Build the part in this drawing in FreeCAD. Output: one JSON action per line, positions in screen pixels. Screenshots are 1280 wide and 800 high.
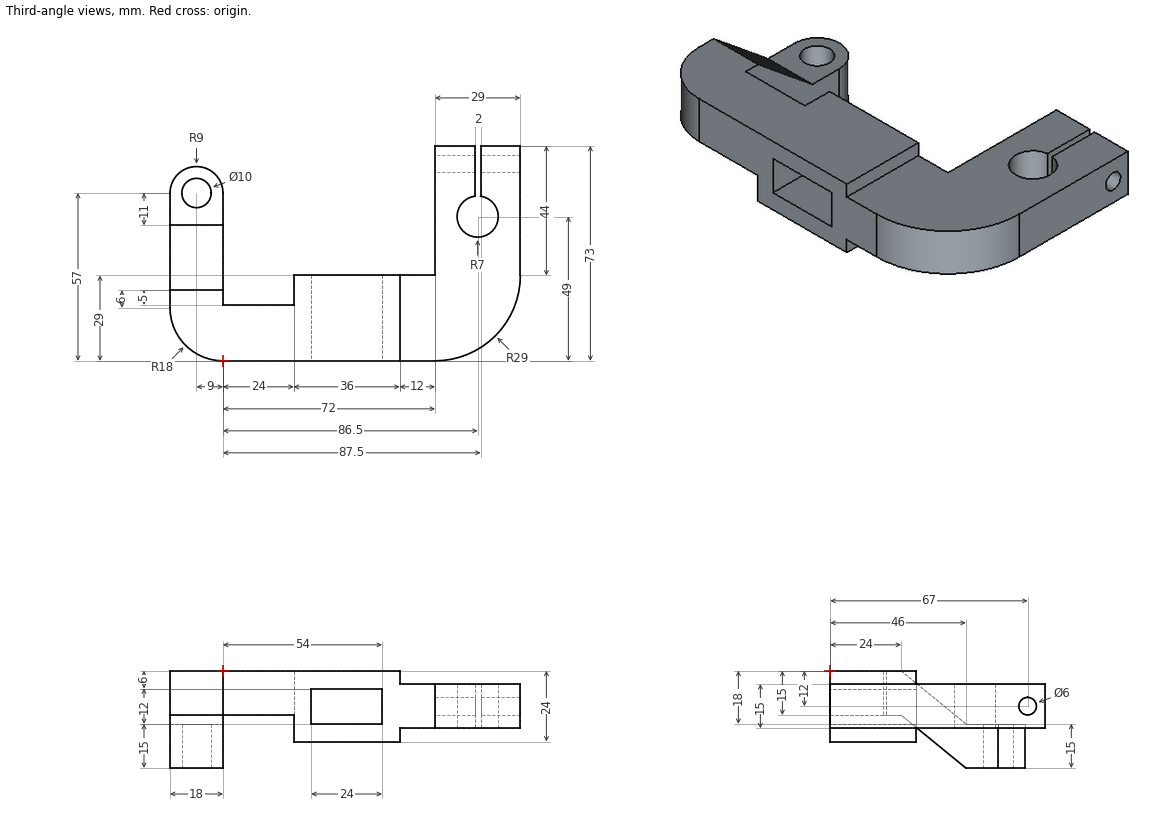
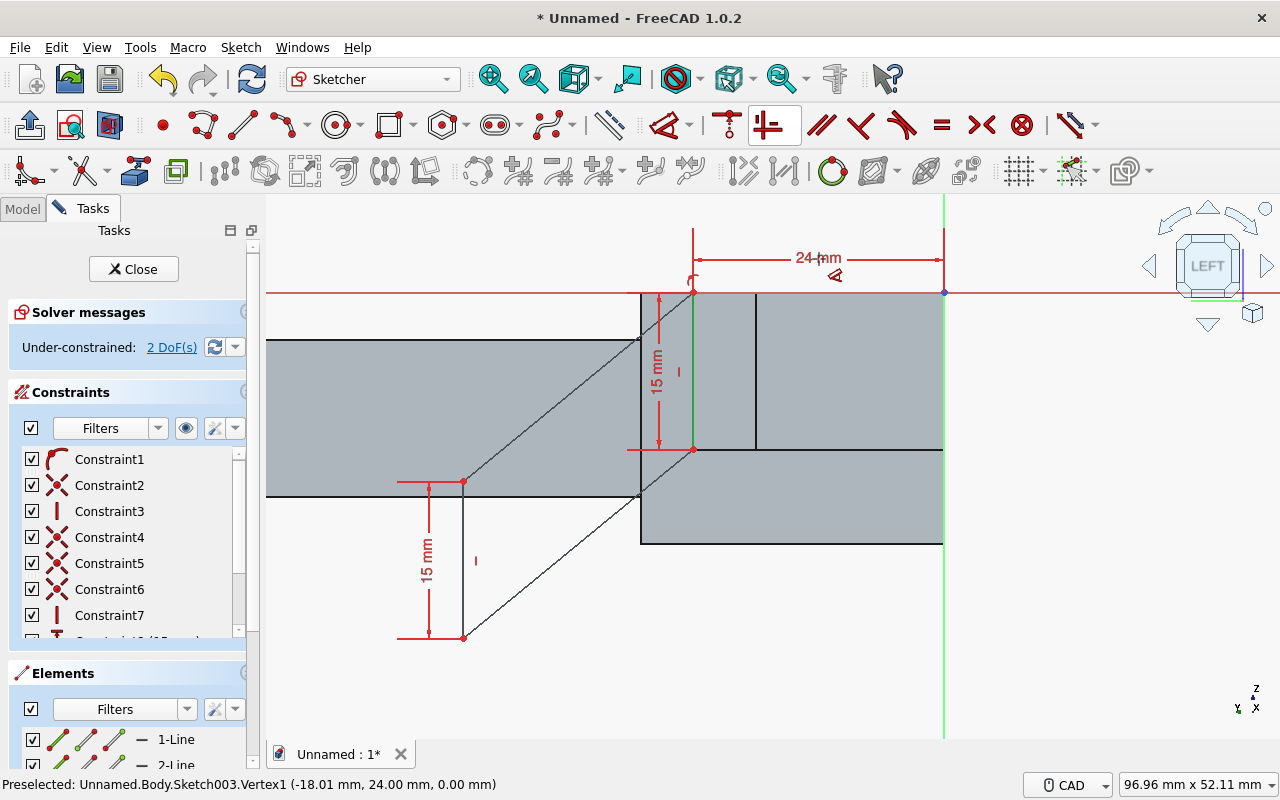
{"action": "left_click", "coordinate": [463, 482]}
{"action": "left_click", "coordinate": [704, 259]}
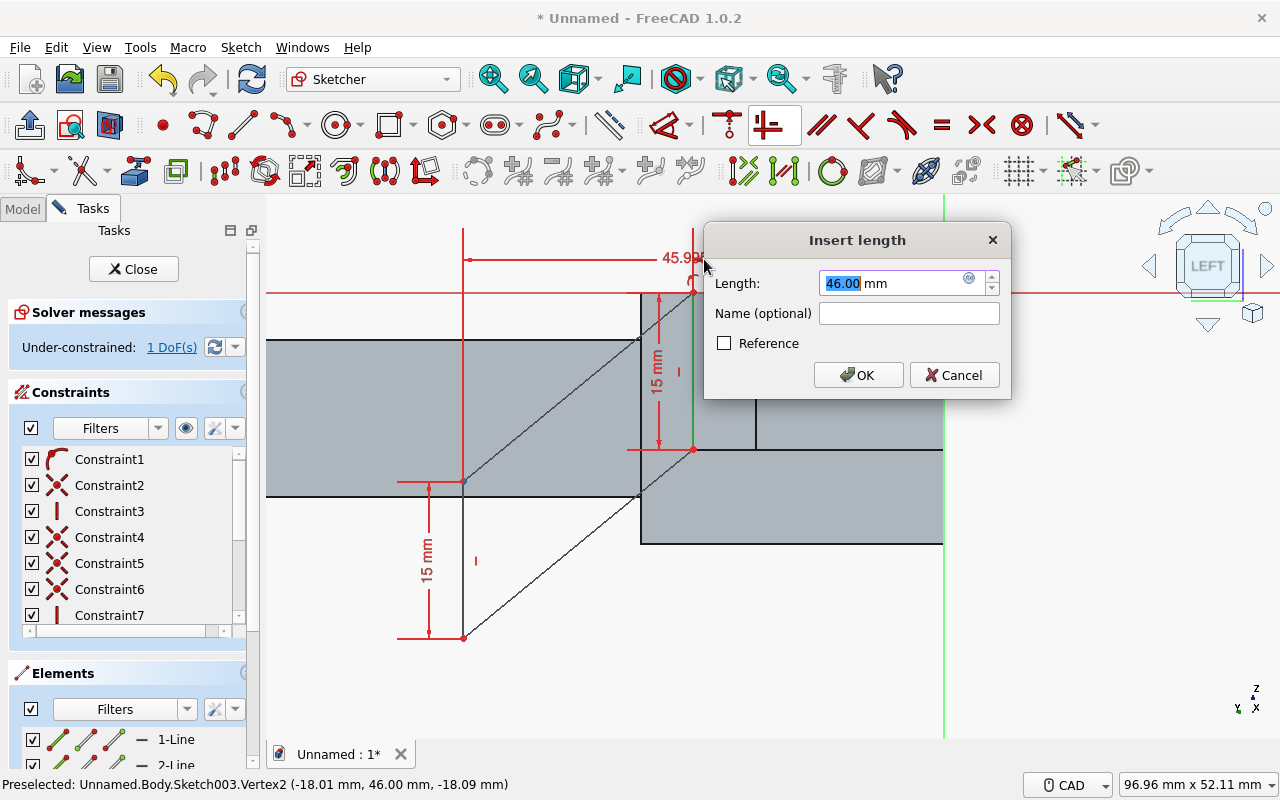
{"action": "type", "text": "46"}
{"action": "key", "text": "Return"}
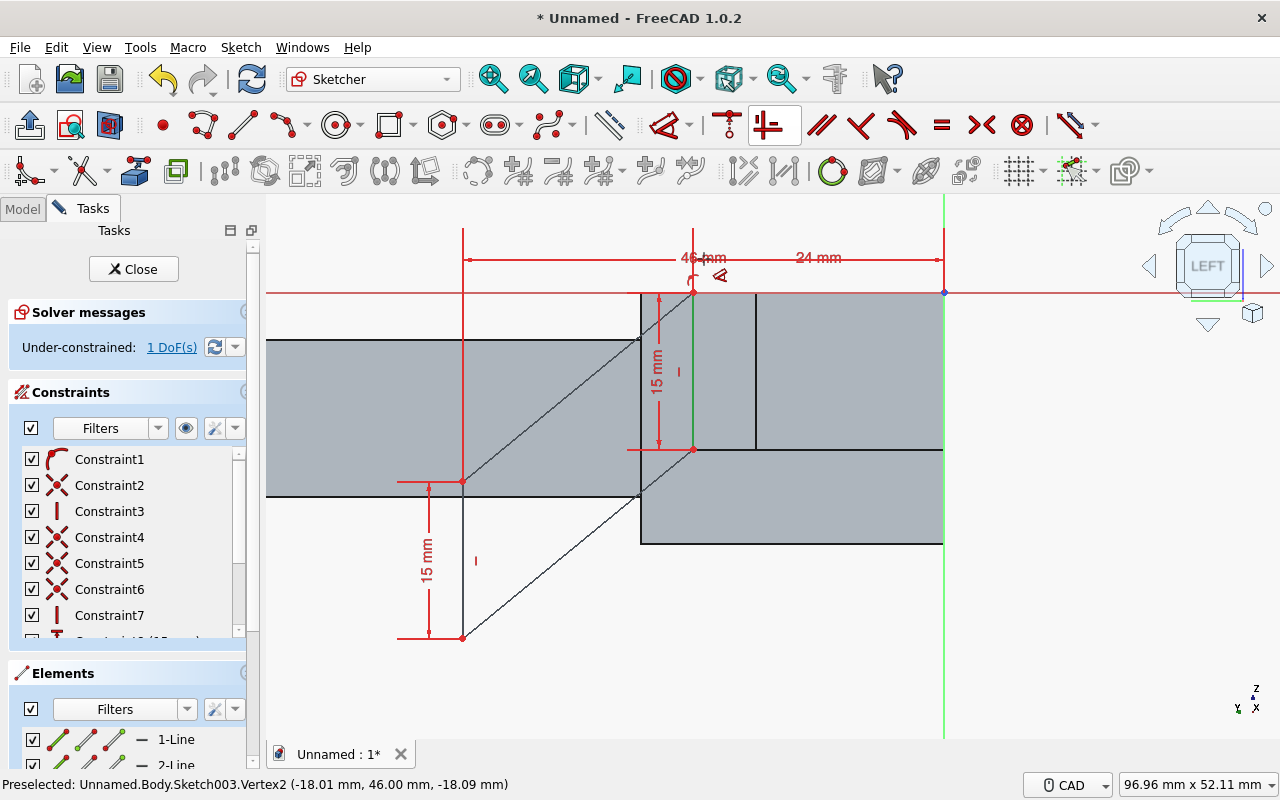
{"action": "left_click", "coordinate": [463, 482]}
{"action": "left_click", "coordinate": [978, 387]}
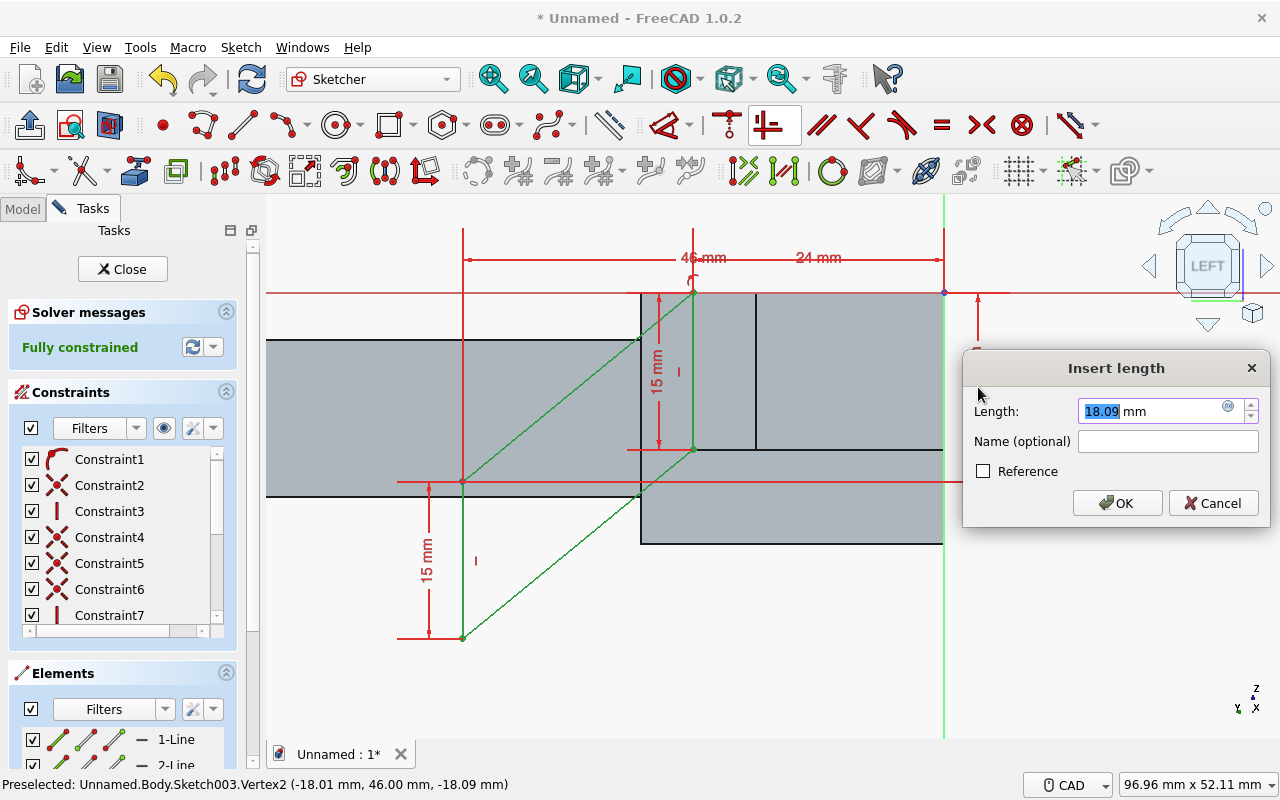
{"action": "type", "text": "18"}
{"action": "key", "text": "Return"}
{"action": "key", "text": "Escape"}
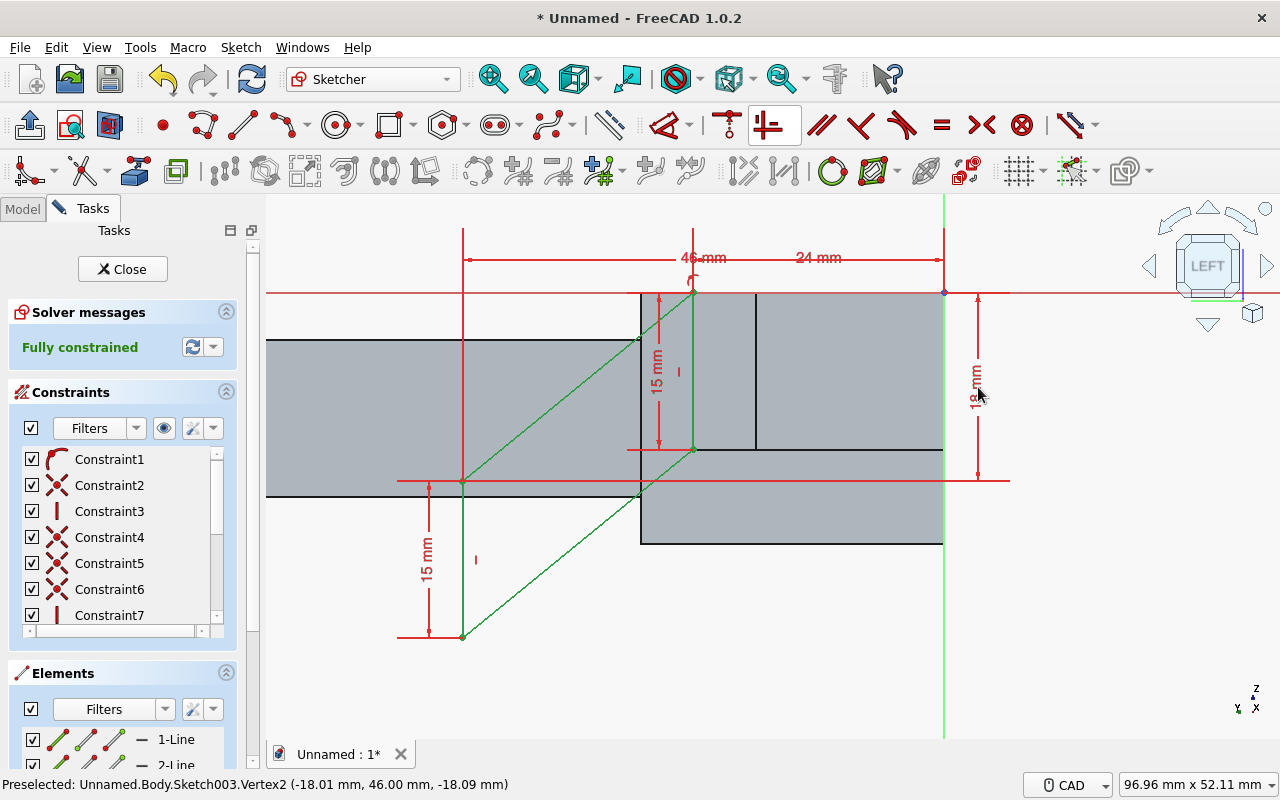
{"action": "left_click", "coordinate": [123, 269]}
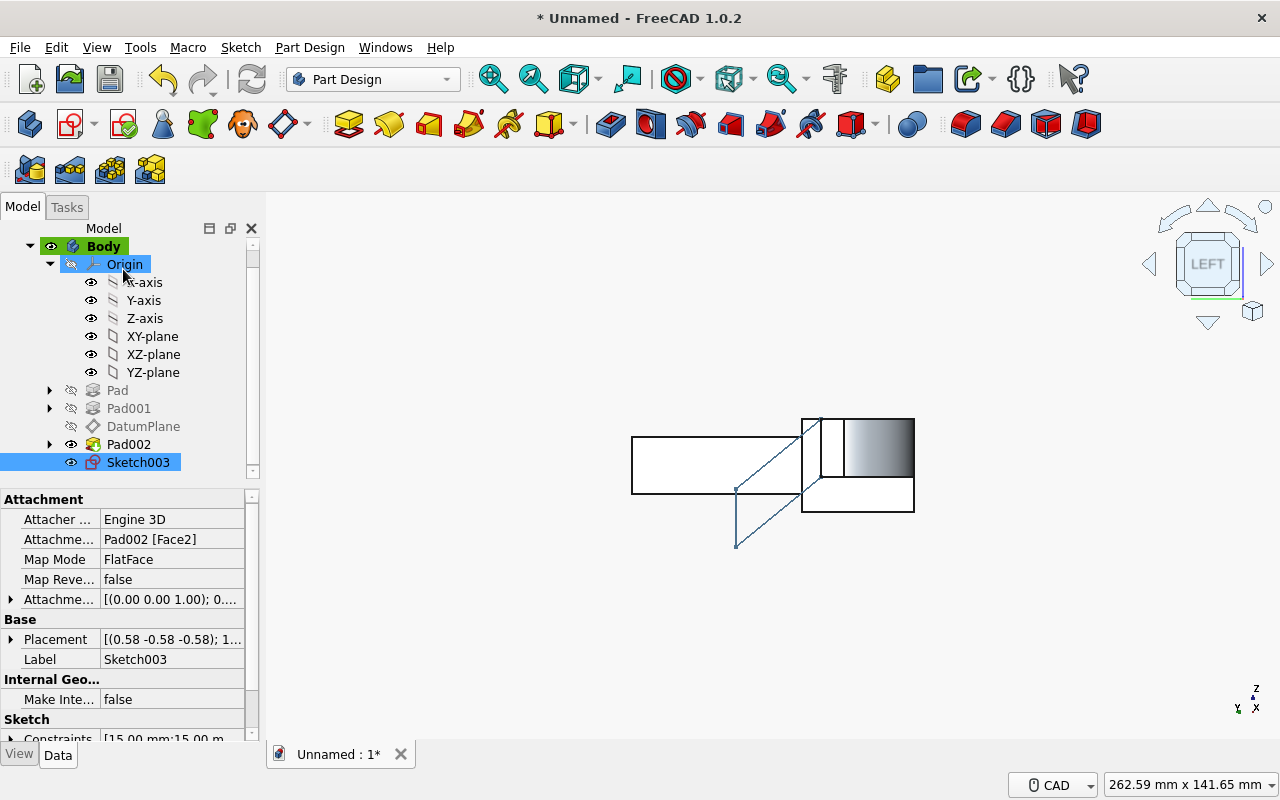
{"action": "left_click", "coordinate": [350, 124]}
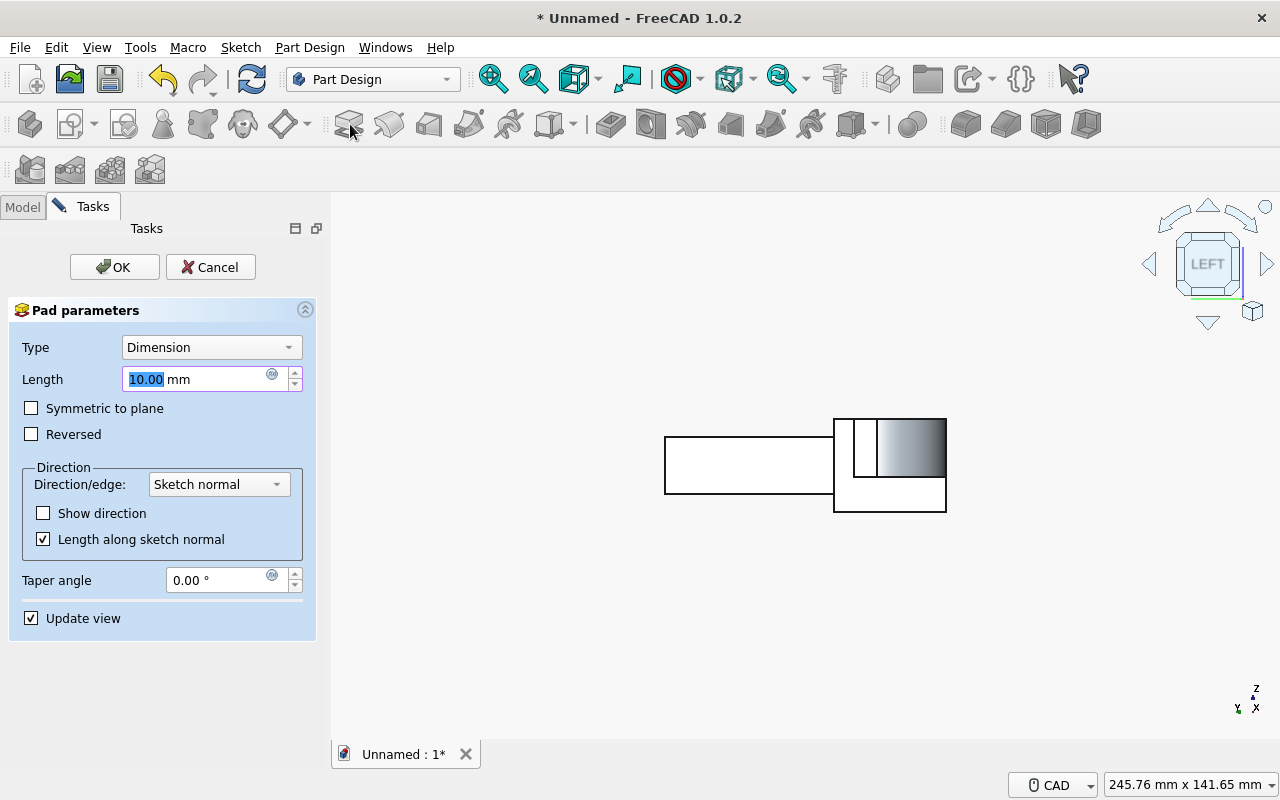
{"action": "type", "text": "18"}
{"action": "key", "text": "Tab"}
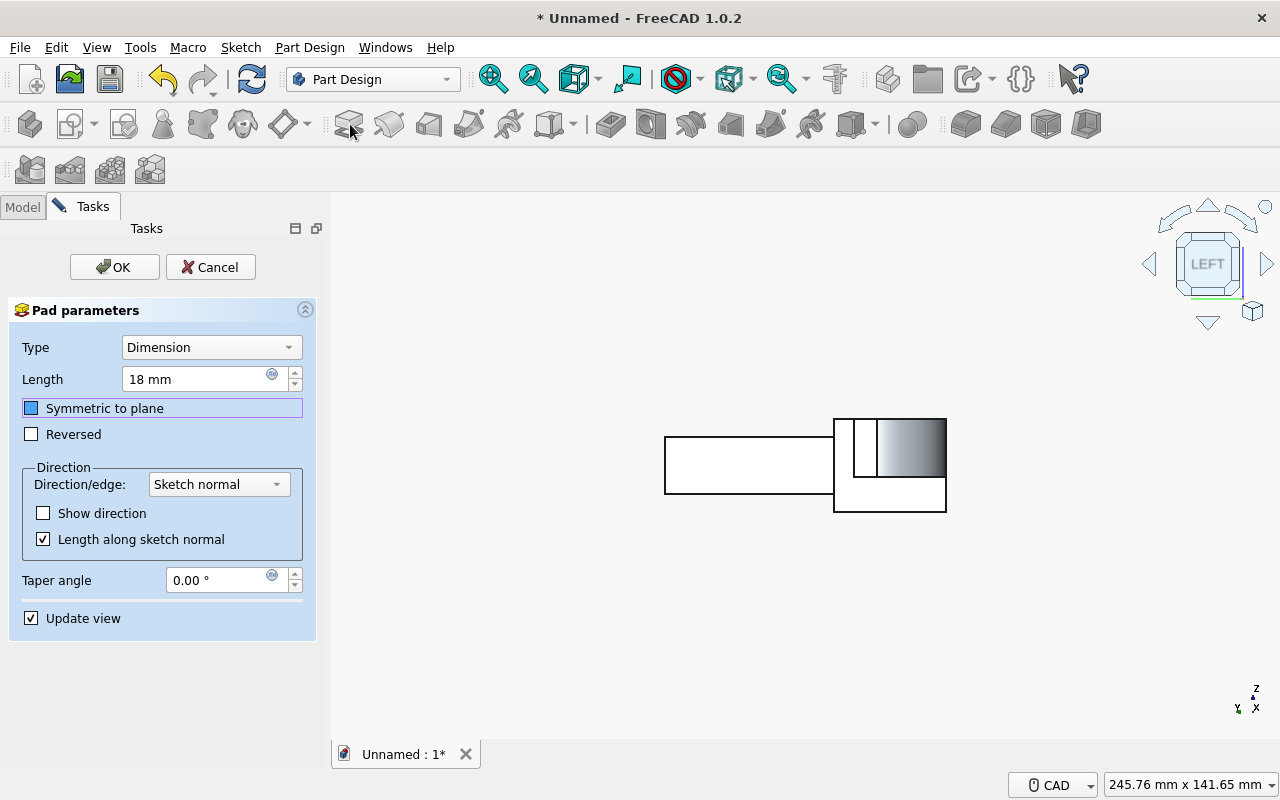
{"action": "left_click", "coordinate": [30, 434]}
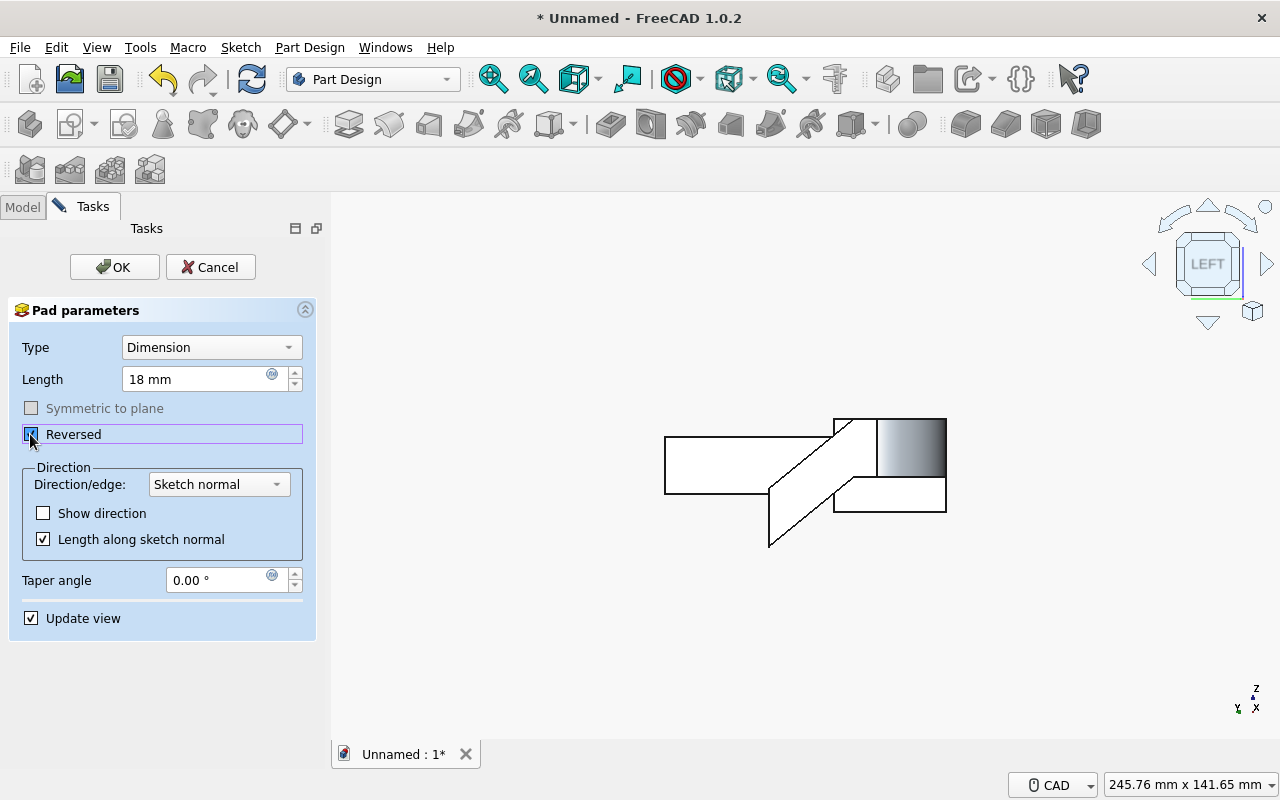
{"action": "left_click", "coordinate": [115, 267]}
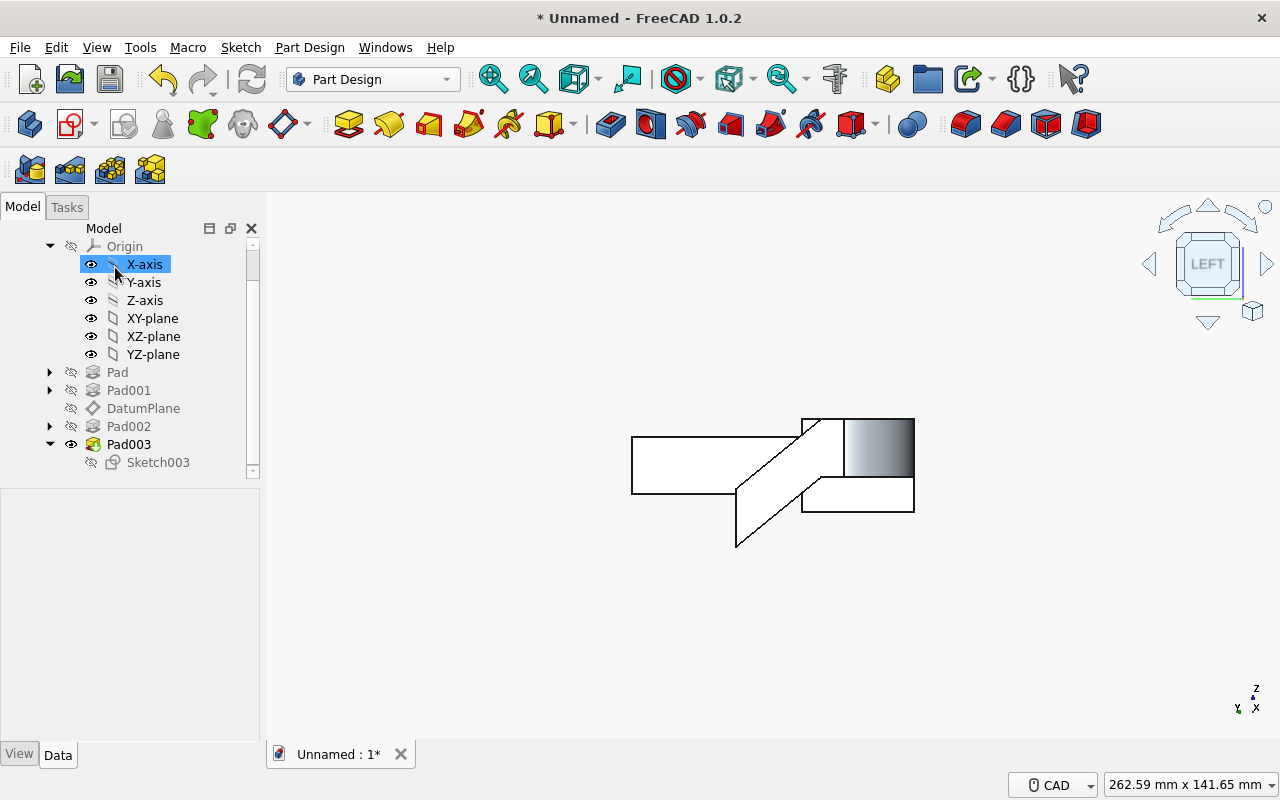
{"action": "left_click", "coordinate": [494, 80]}